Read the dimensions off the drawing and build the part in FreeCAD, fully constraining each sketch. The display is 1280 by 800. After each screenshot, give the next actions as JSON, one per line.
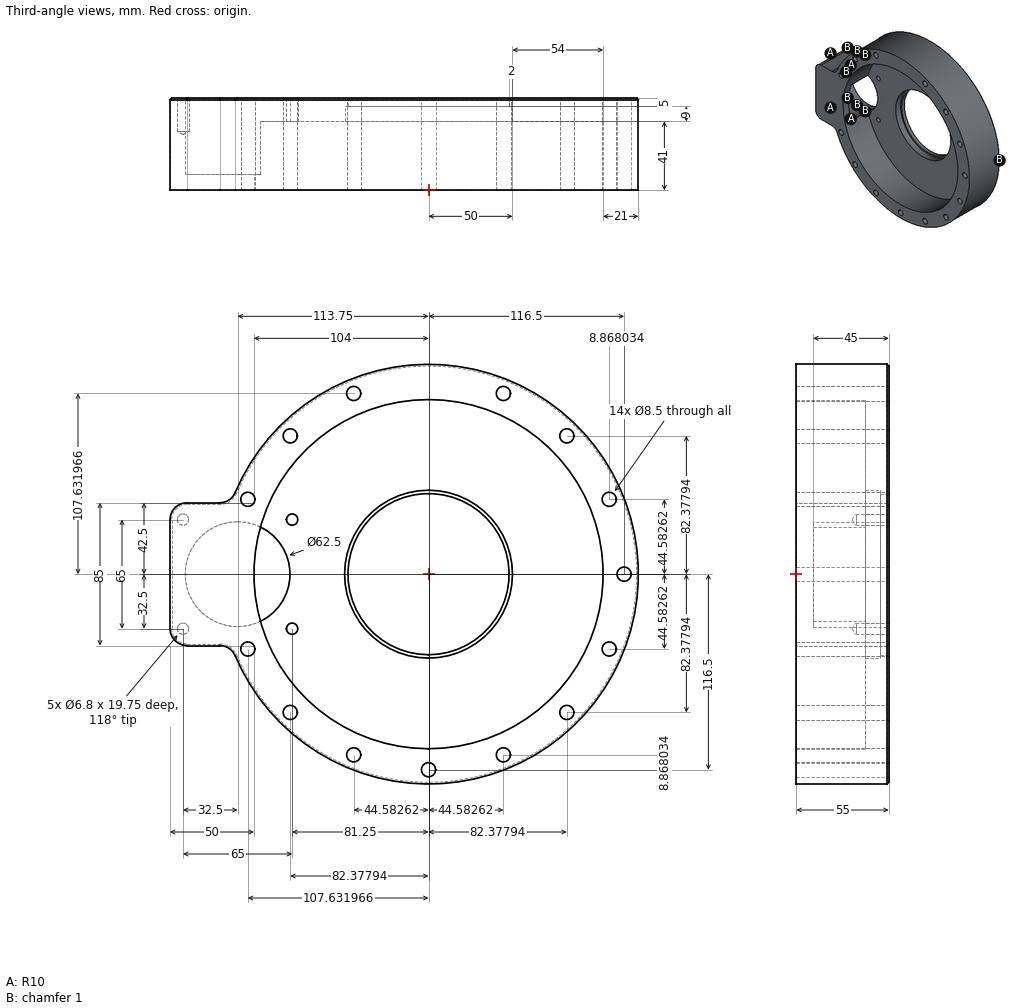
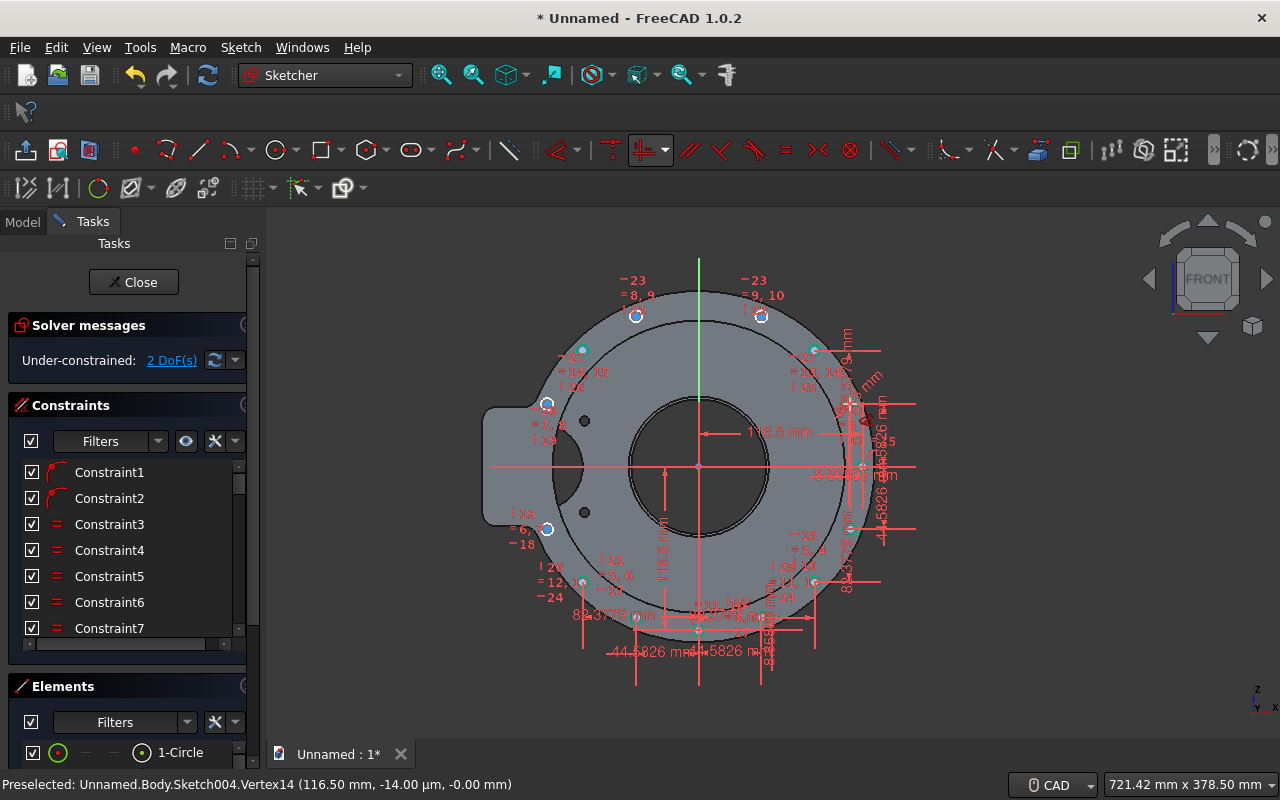
{"action": "left_click", "coordinate": [547, 529]}
{"action": "left_click", "coordinate": [588, 563]}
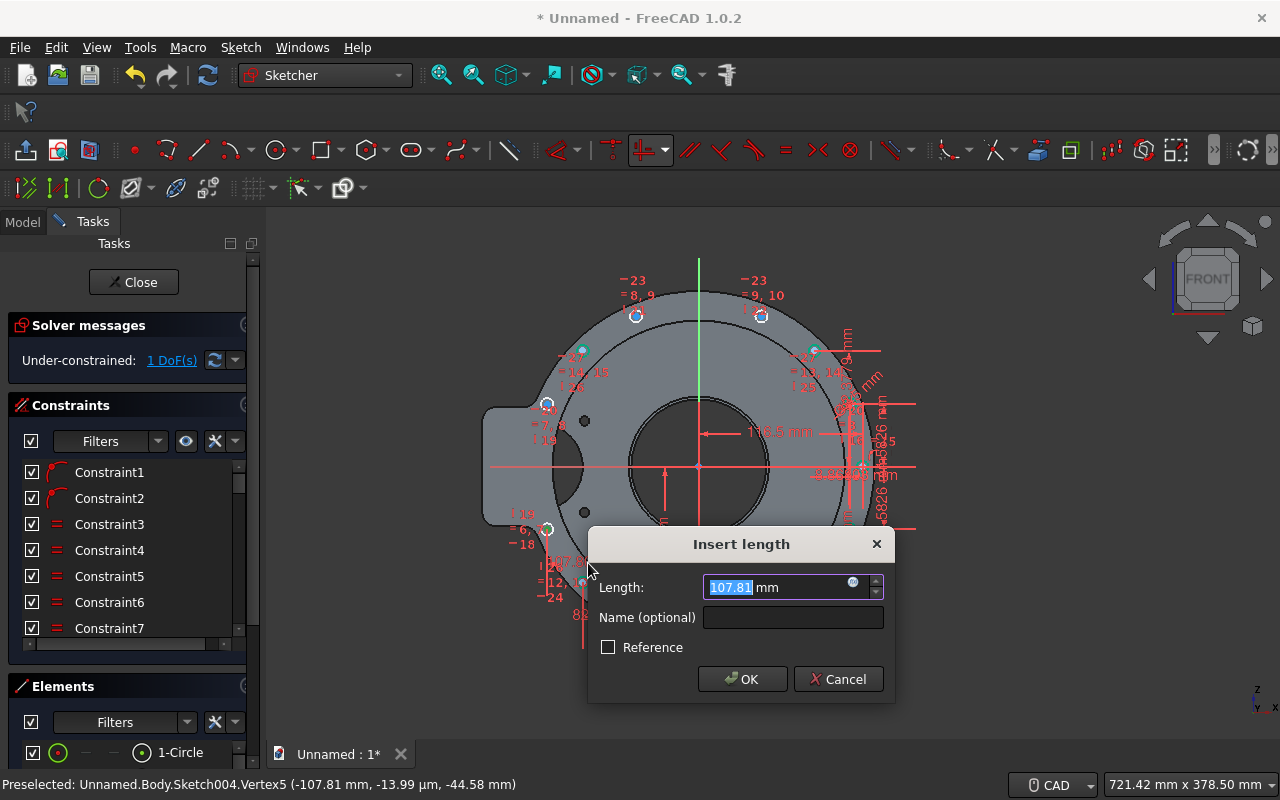
{"action": "type", "text": "107.631966"}
{"action": "key", "text": "Return"}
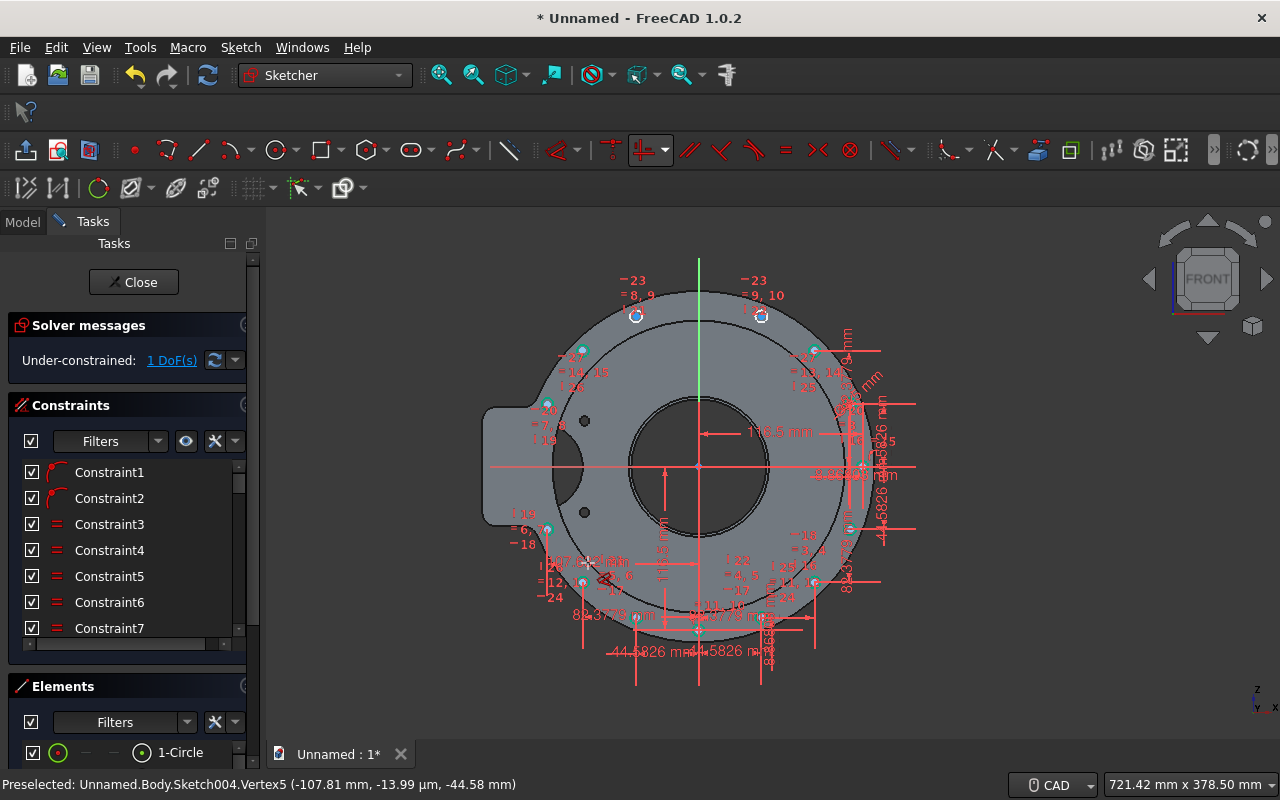
{"action": "left_click", "coordinate": [636, 316]}
{"action": "left_click", "coordinate": [602, 392]}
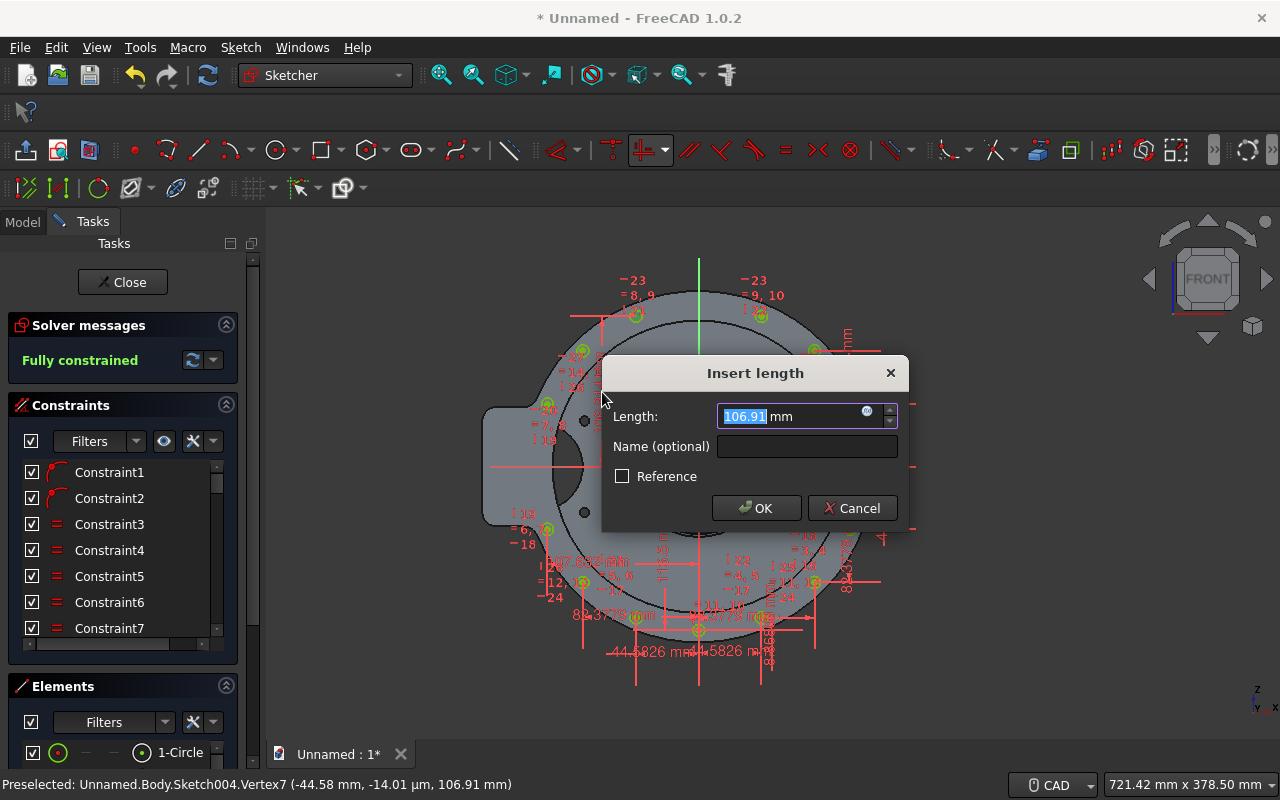
{"action": "type", "text": "107.631966"}
{"action": "key", "text": "Return"}
{"action": "key", "text": "Escape"}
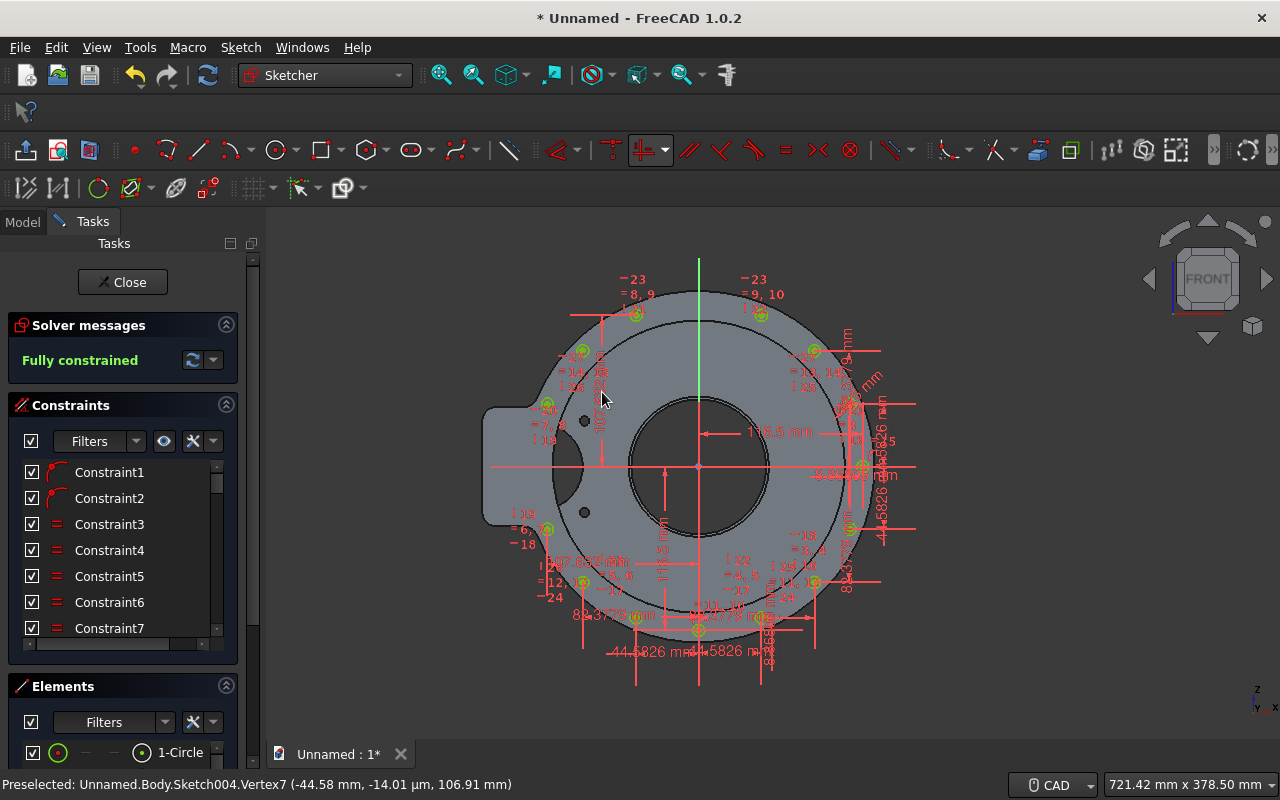
{"action": "left_click", "coordinate": [123, 282]}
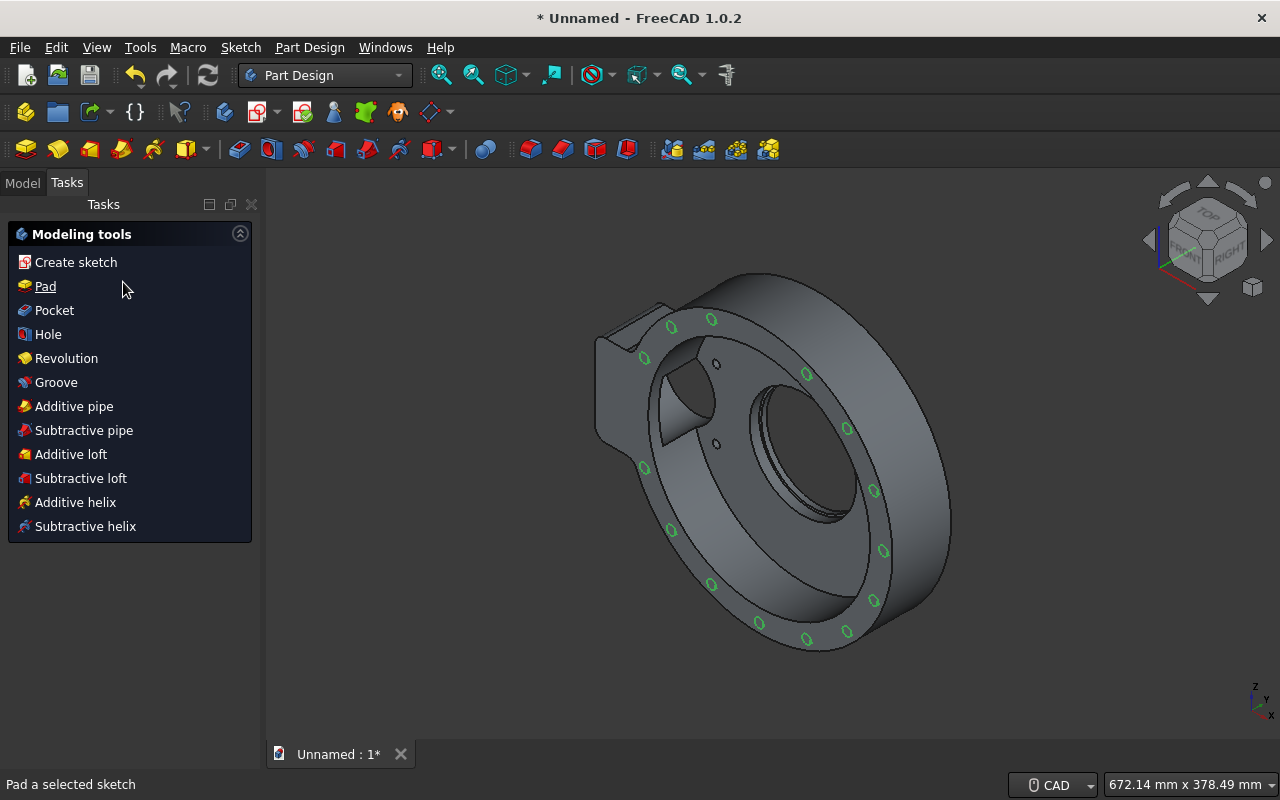
{"action": "left_click", "coordinate": [272, 150]}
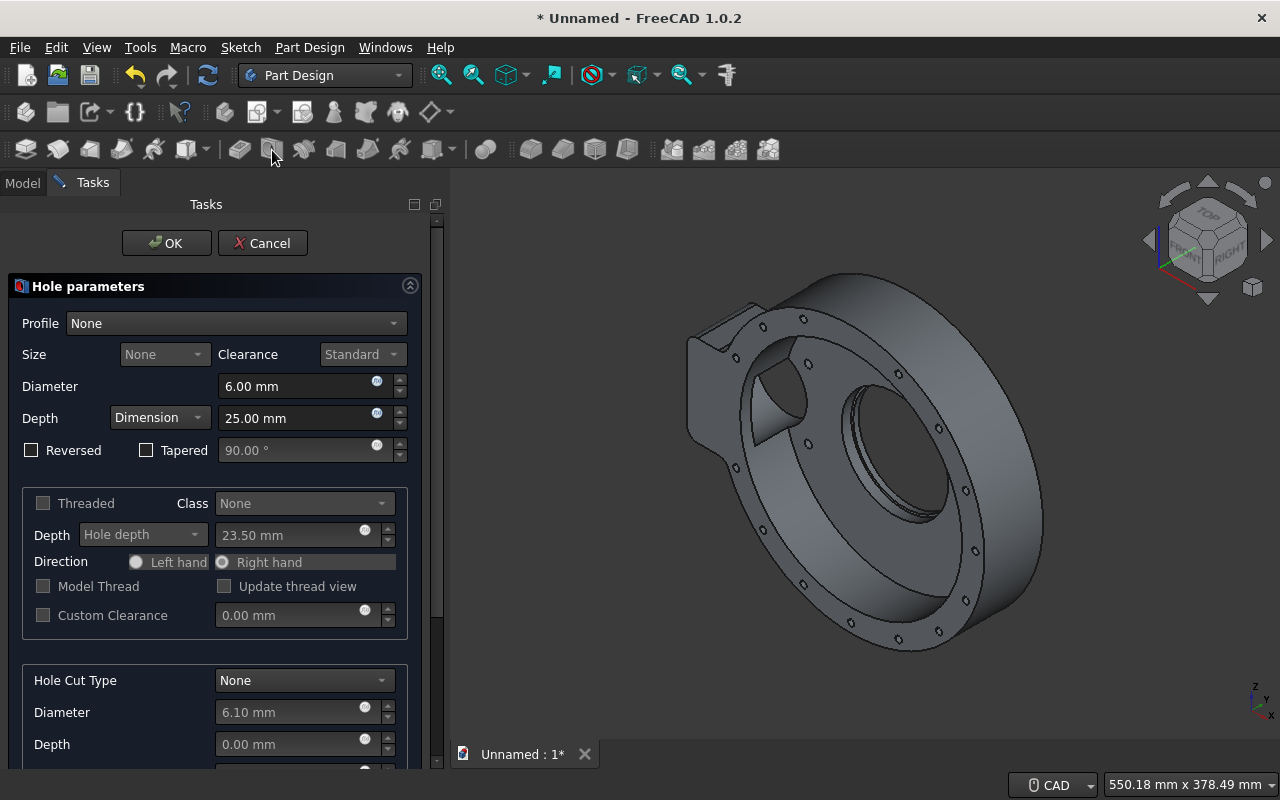
{"action": "triple_click", "coordinate": [305, 386]}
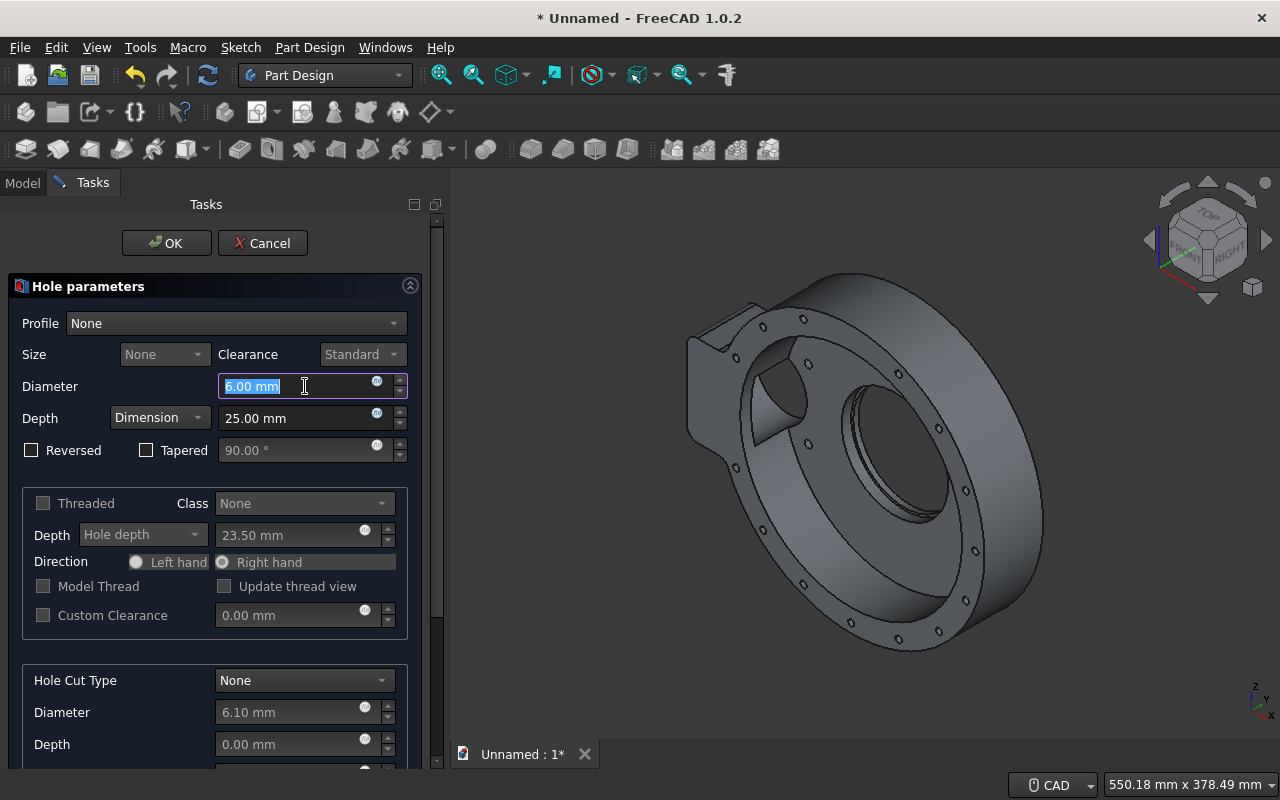
{"action": "type", "text": "8.5"}
{"action": "key", "text": "Tab"}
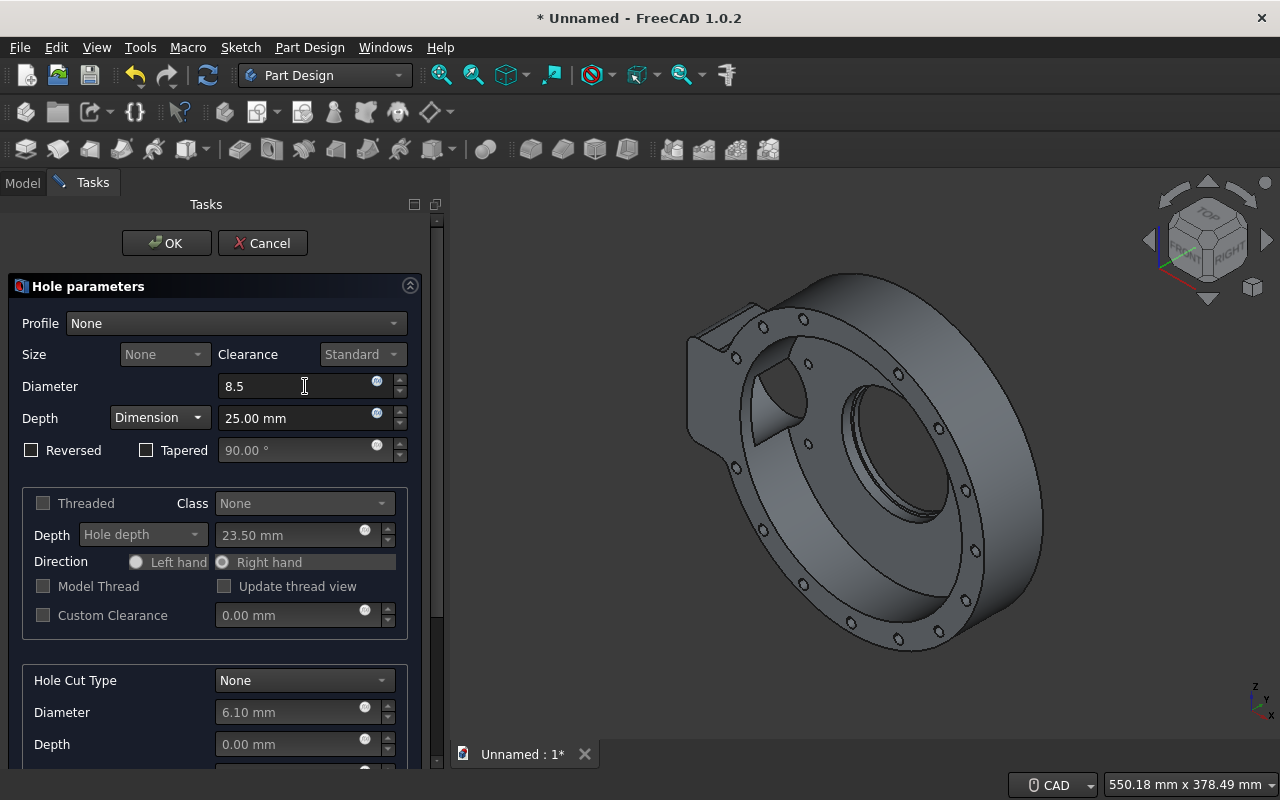
{"action": "left_click", "coordinate": [161, 418]}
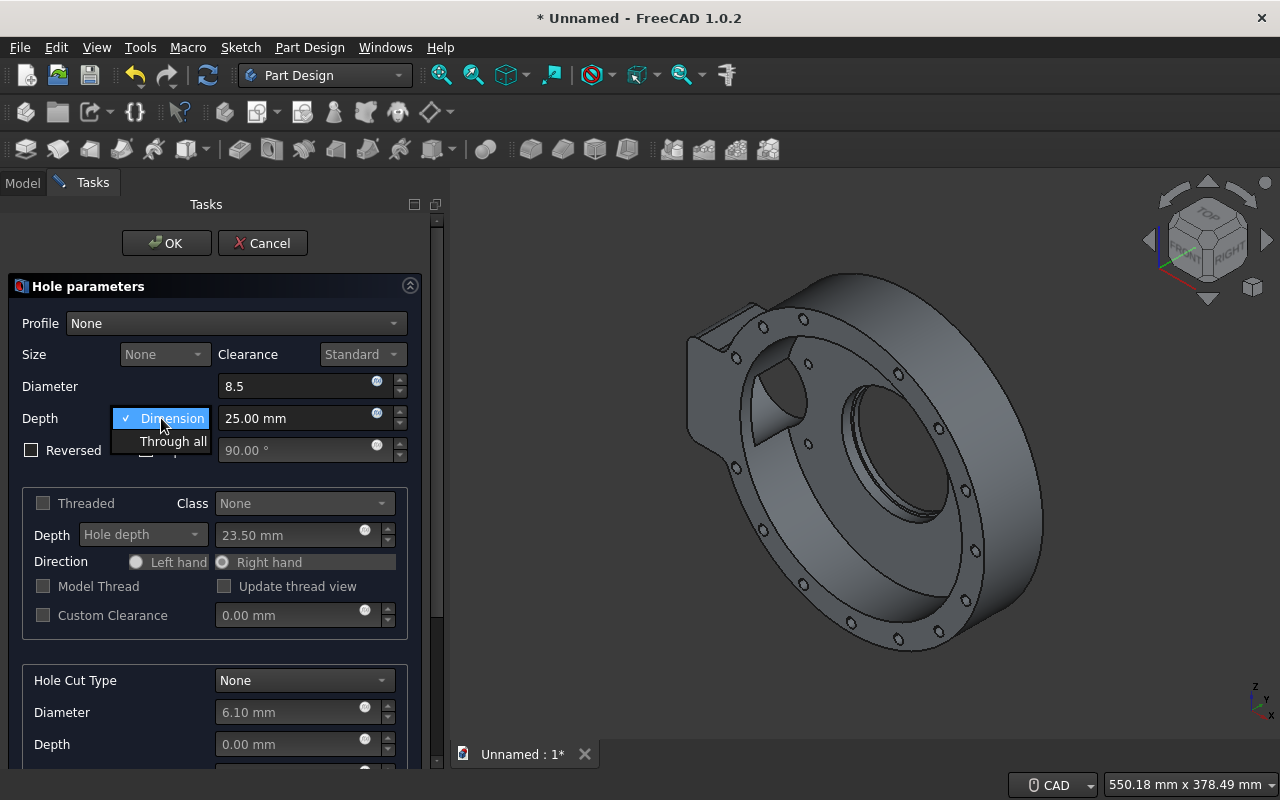
{"action": "left_click", "coordinate": [160, 442]}